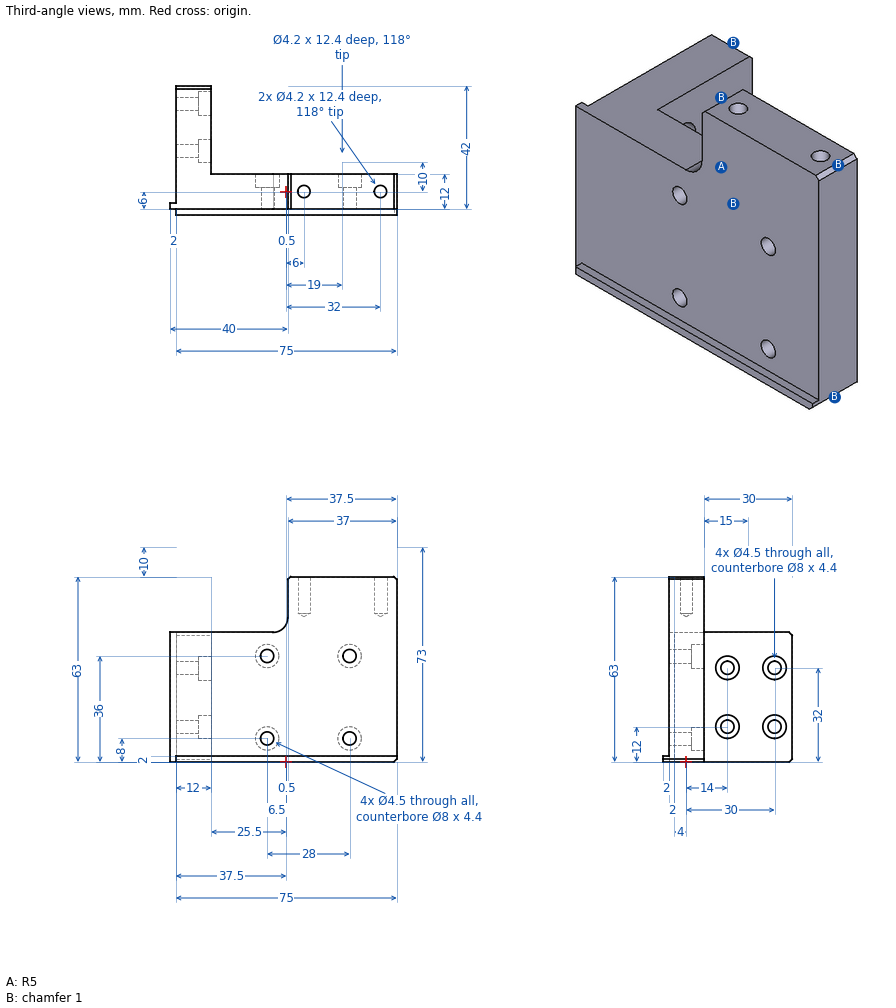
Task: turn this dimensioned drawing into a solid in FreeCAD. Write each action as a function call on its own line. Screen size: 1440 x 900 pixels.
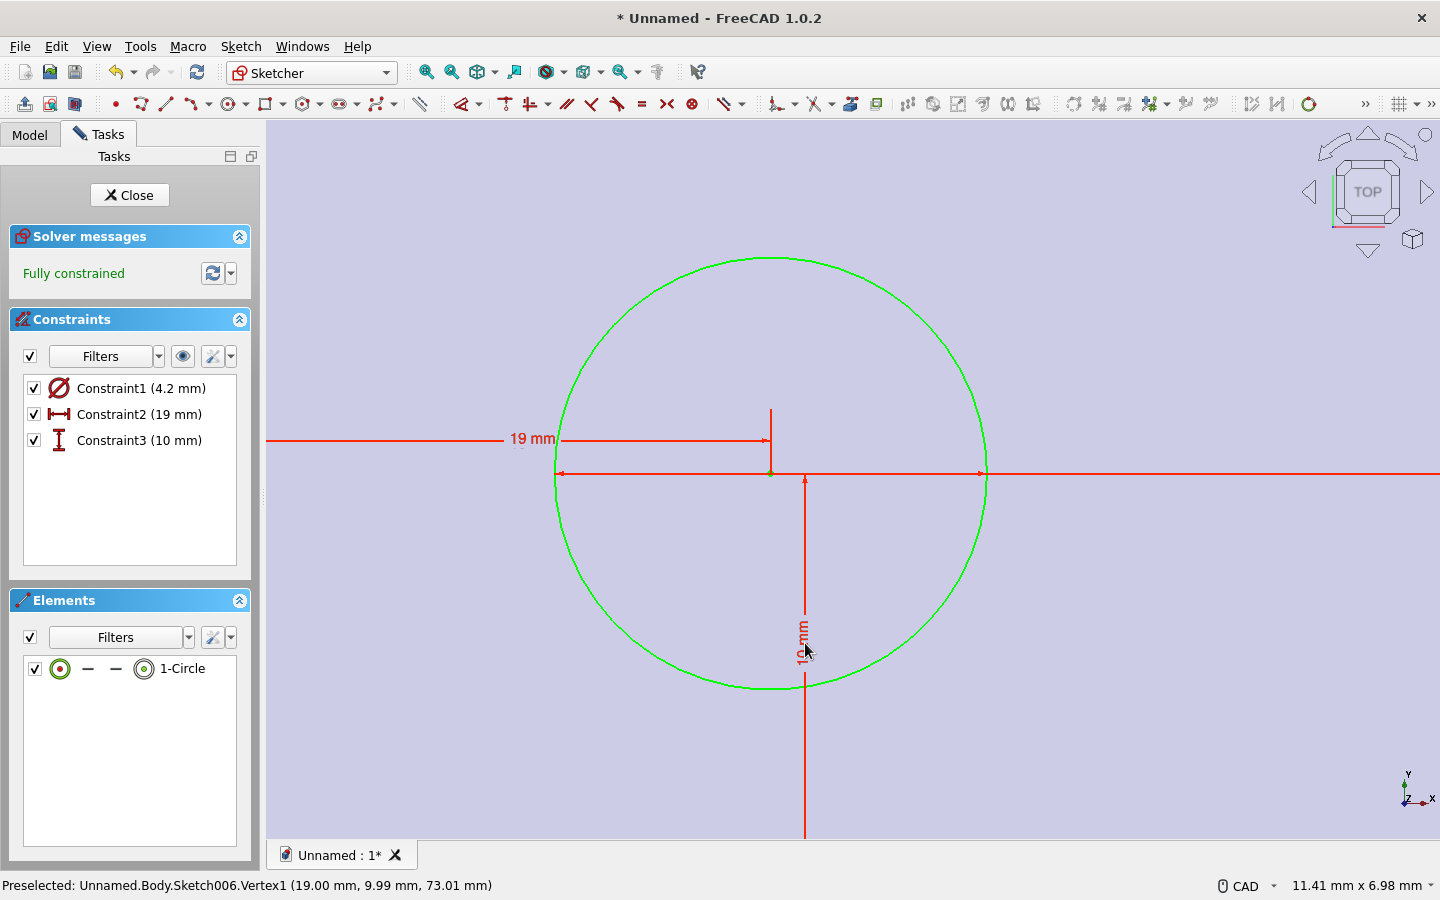
click(130, 195)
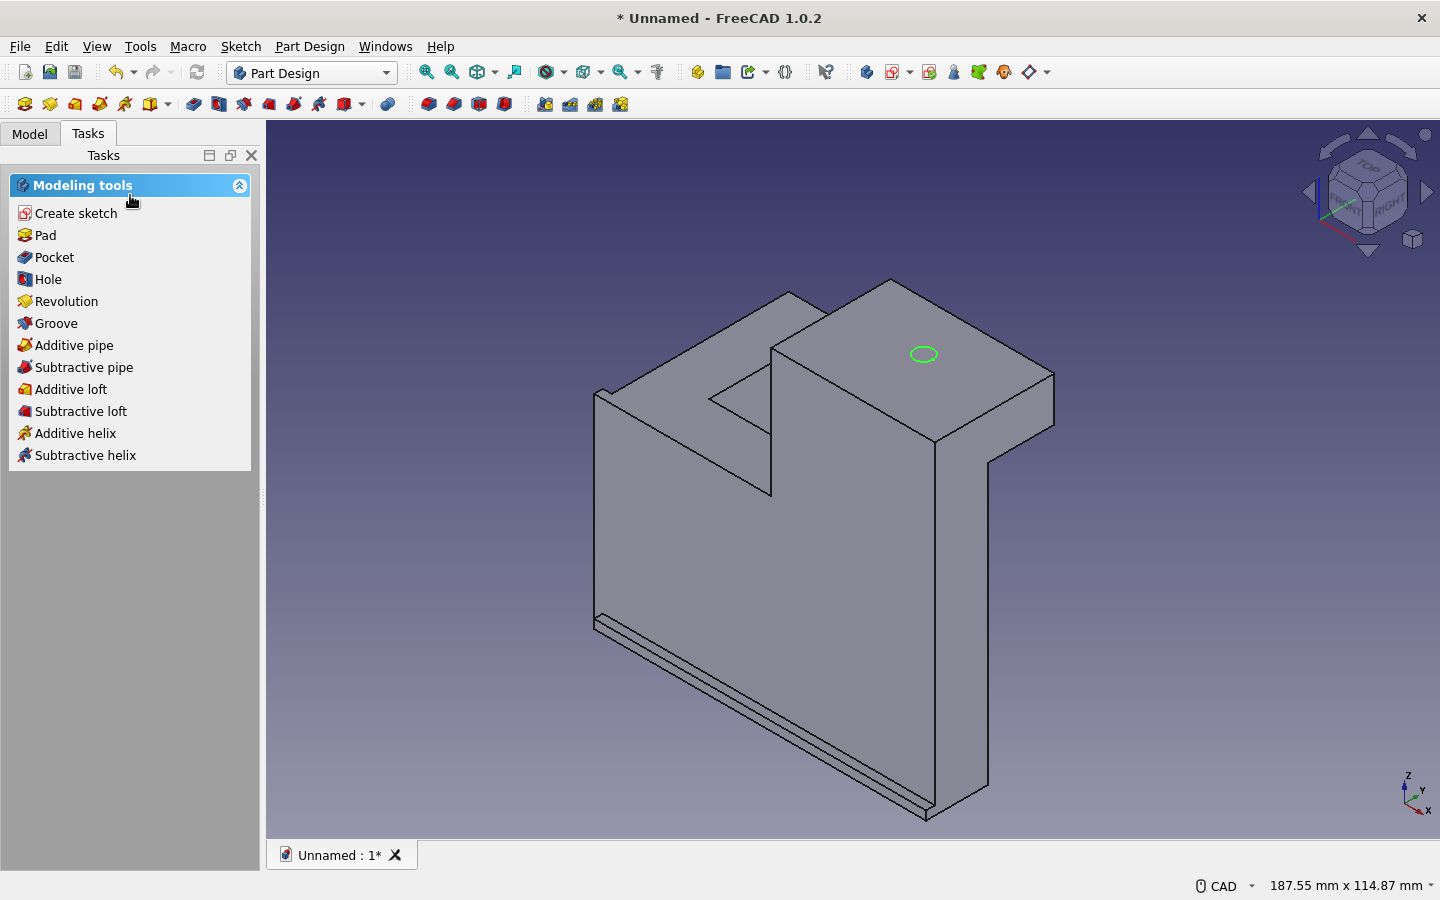
click(219, 104)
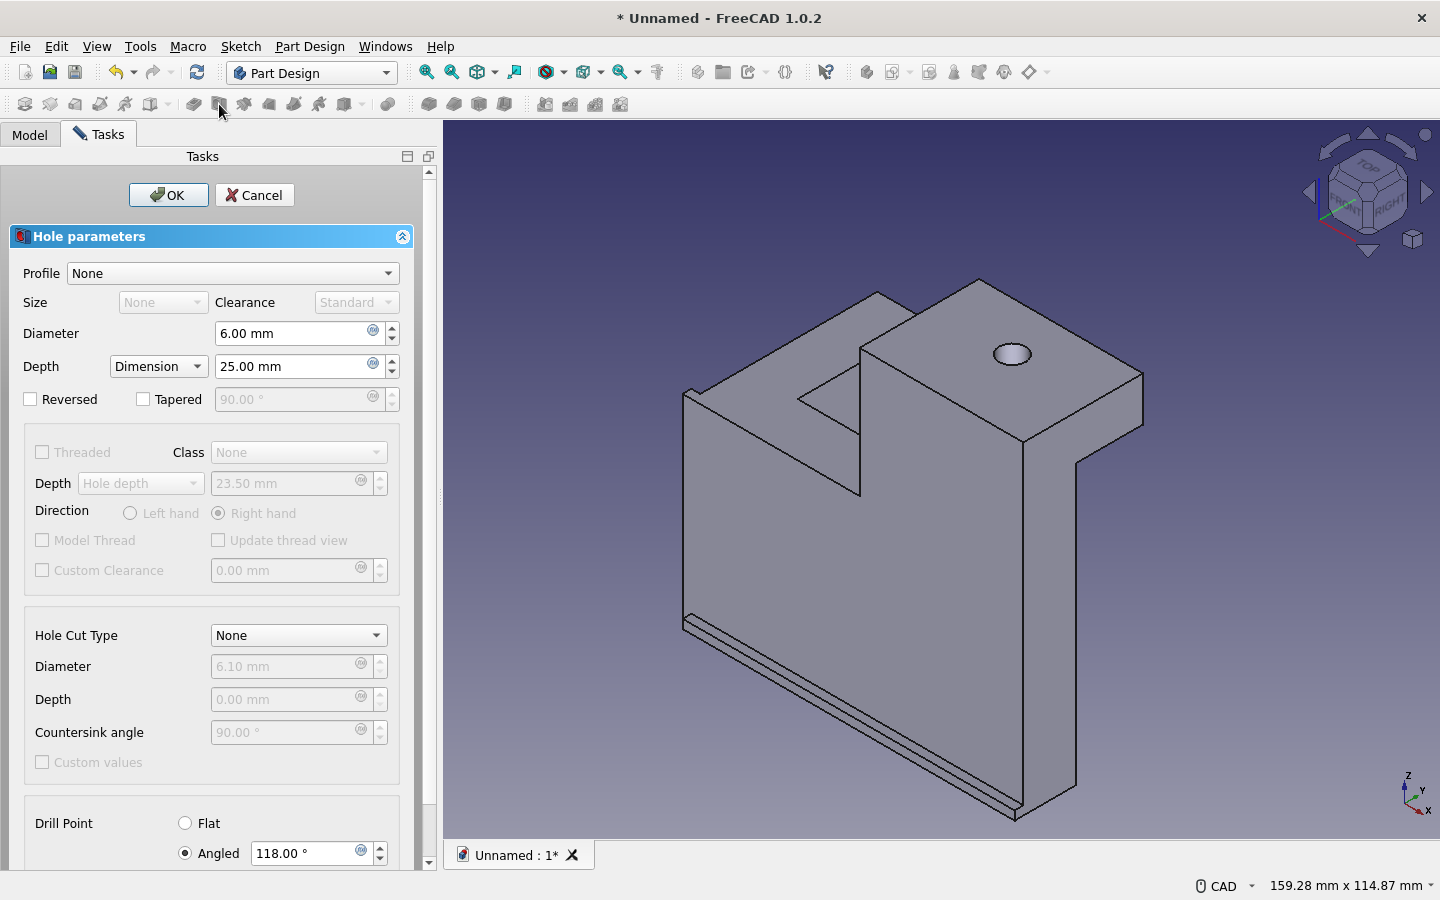
triple_click(300, 334)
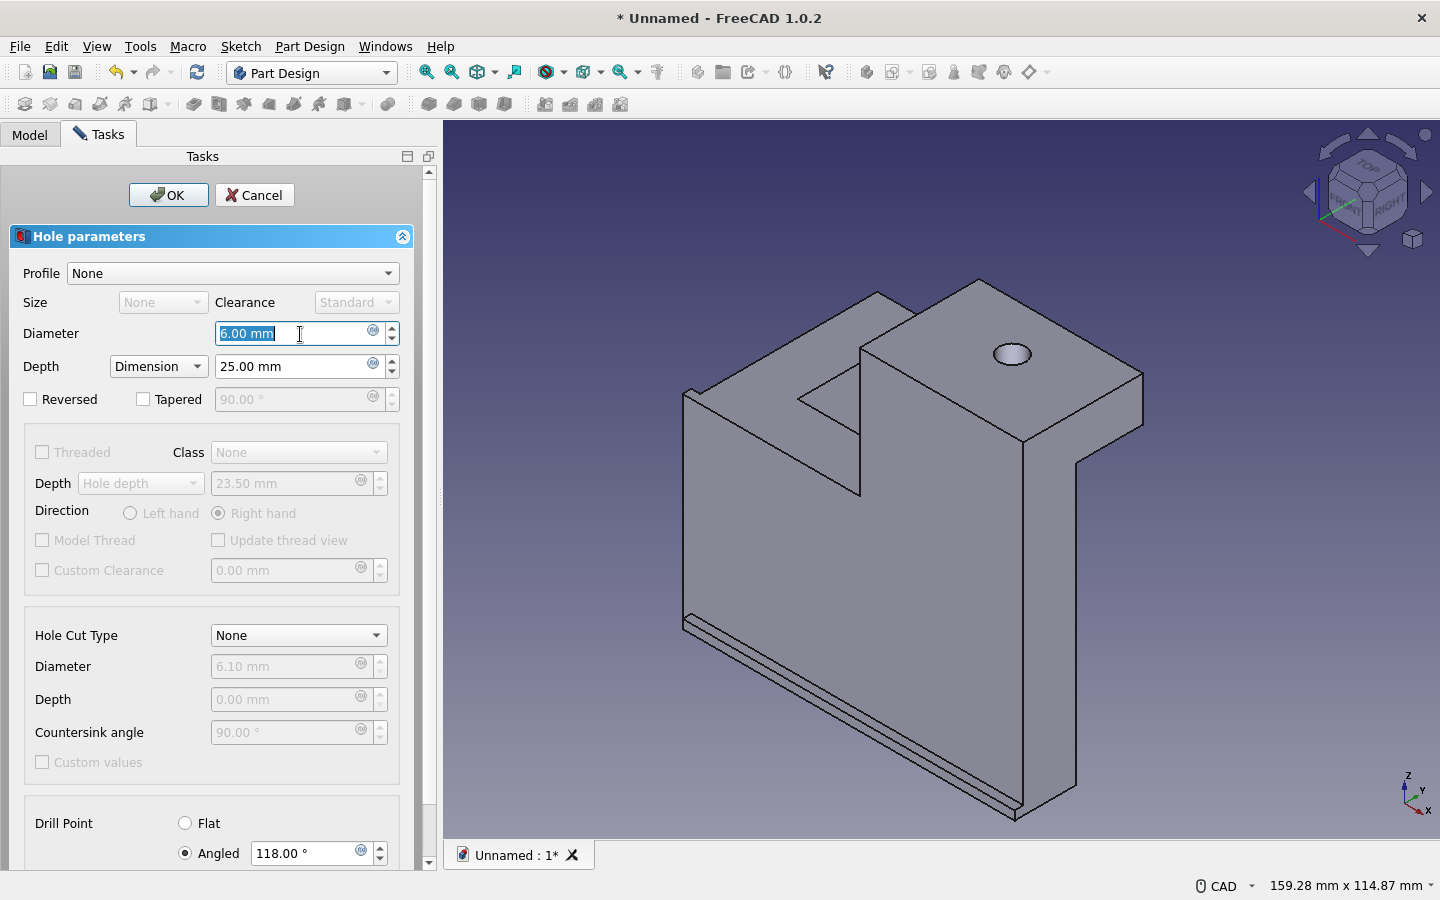
text(4.2)
key(Tab)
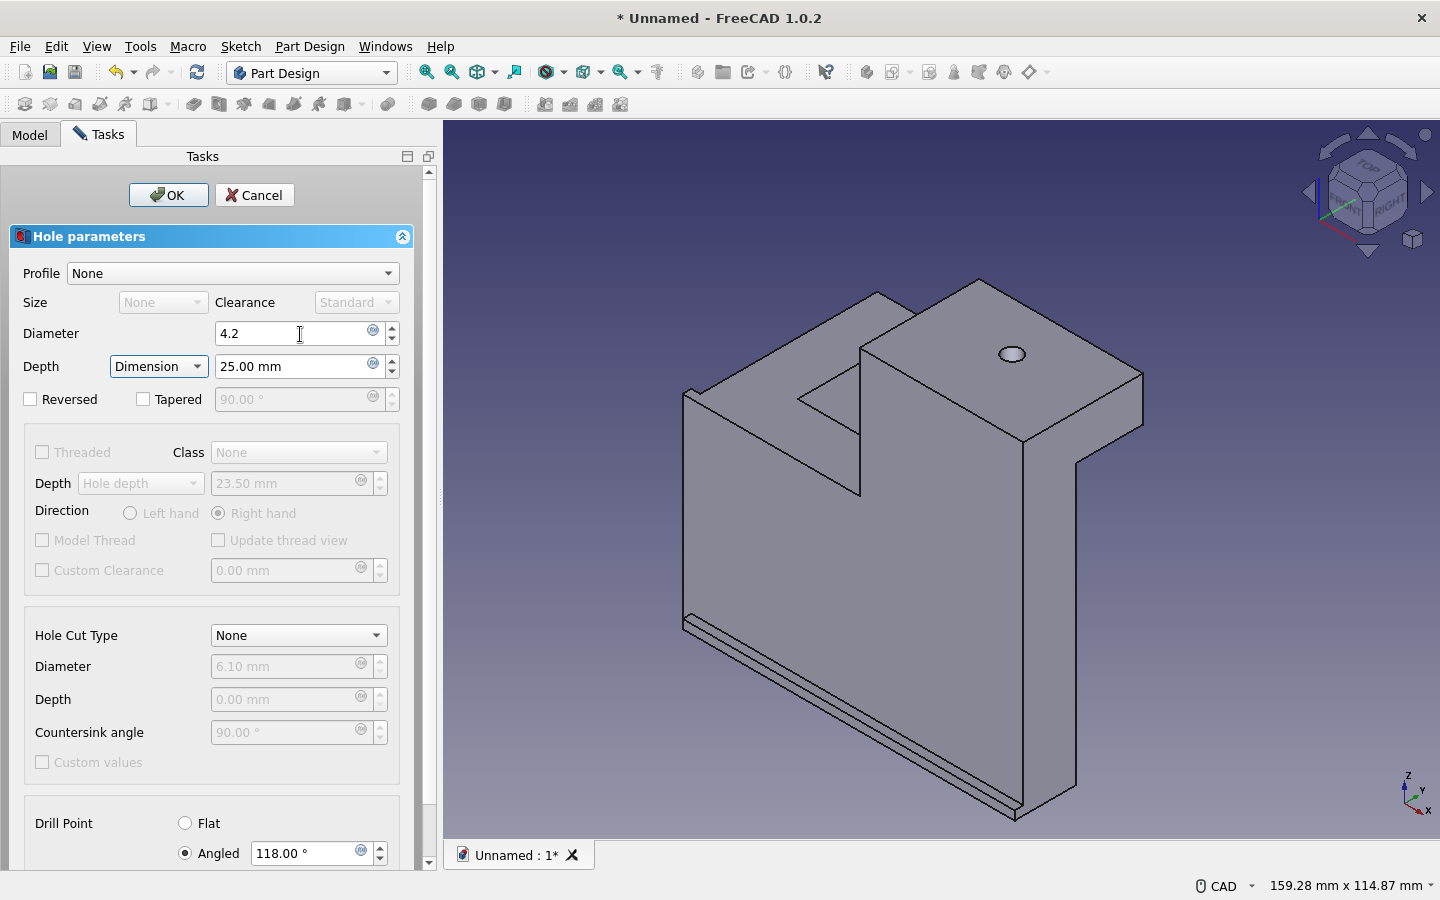
triple_click(300, 366)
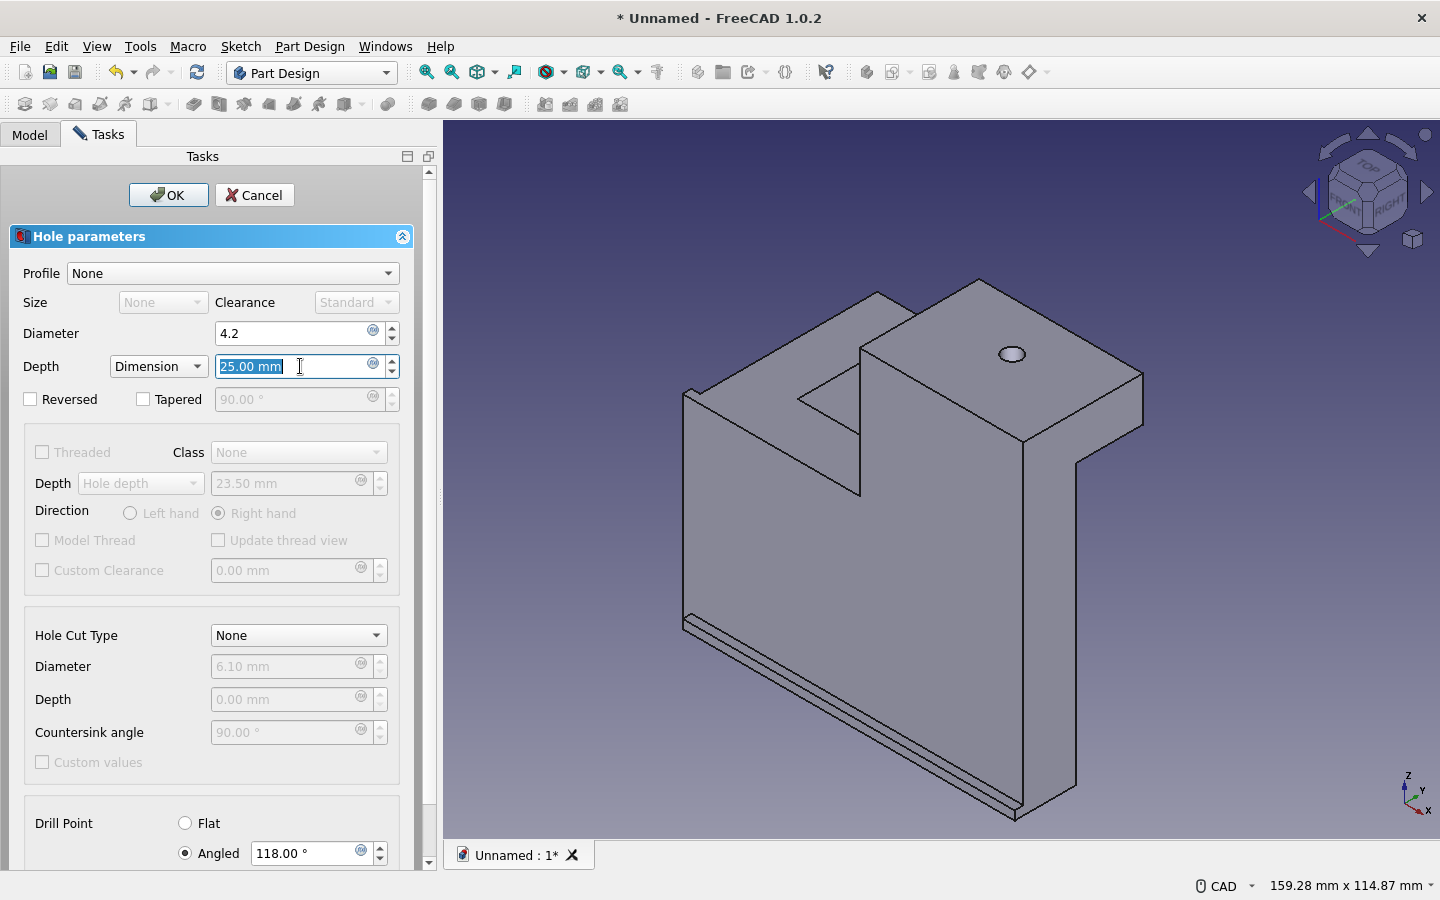
text(12.4)
key(Tab)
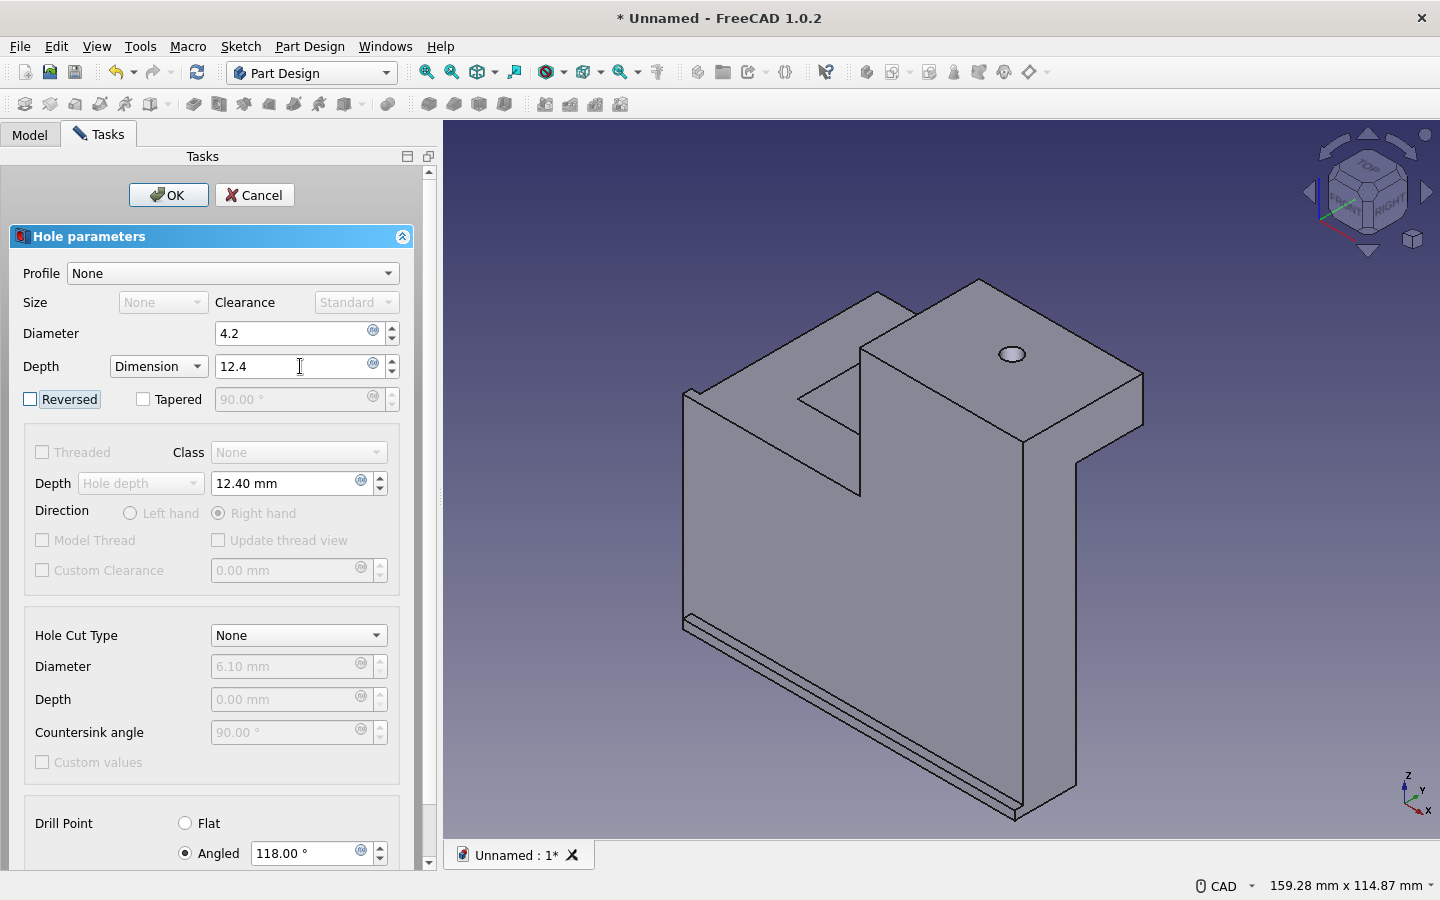
click(169, 195)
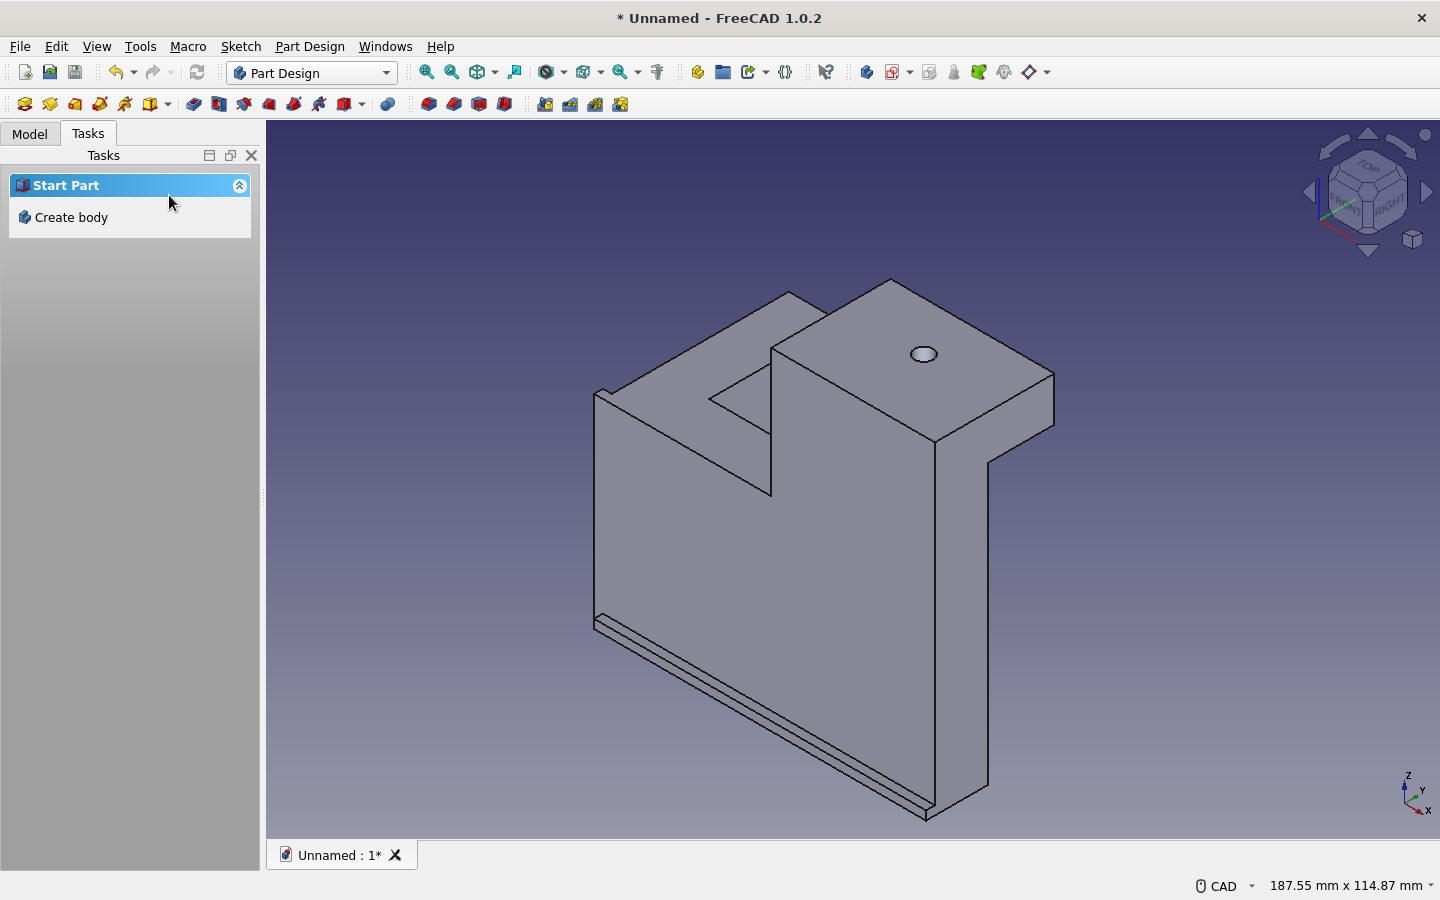
key(3)